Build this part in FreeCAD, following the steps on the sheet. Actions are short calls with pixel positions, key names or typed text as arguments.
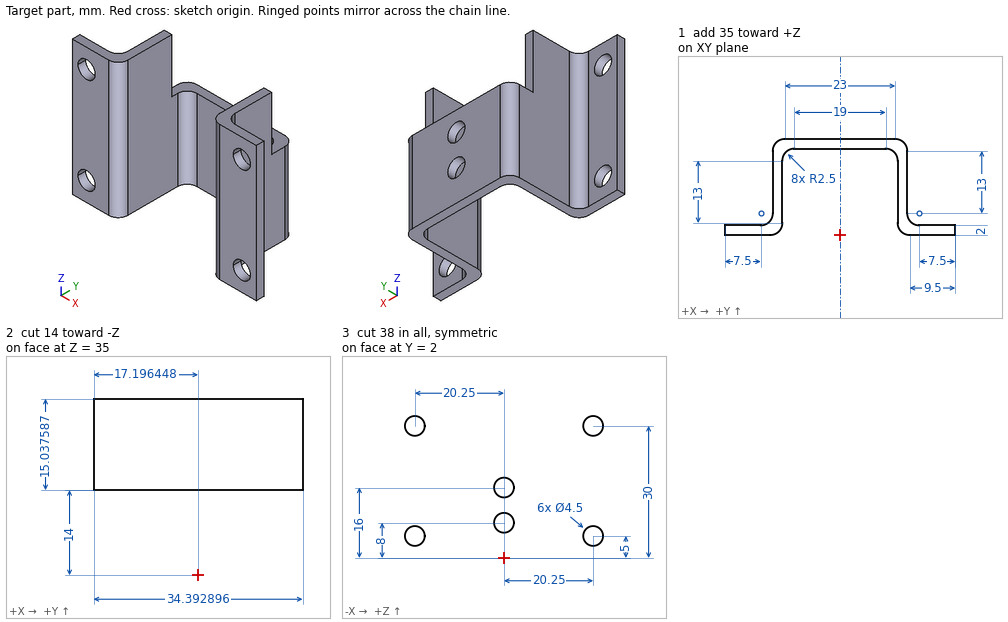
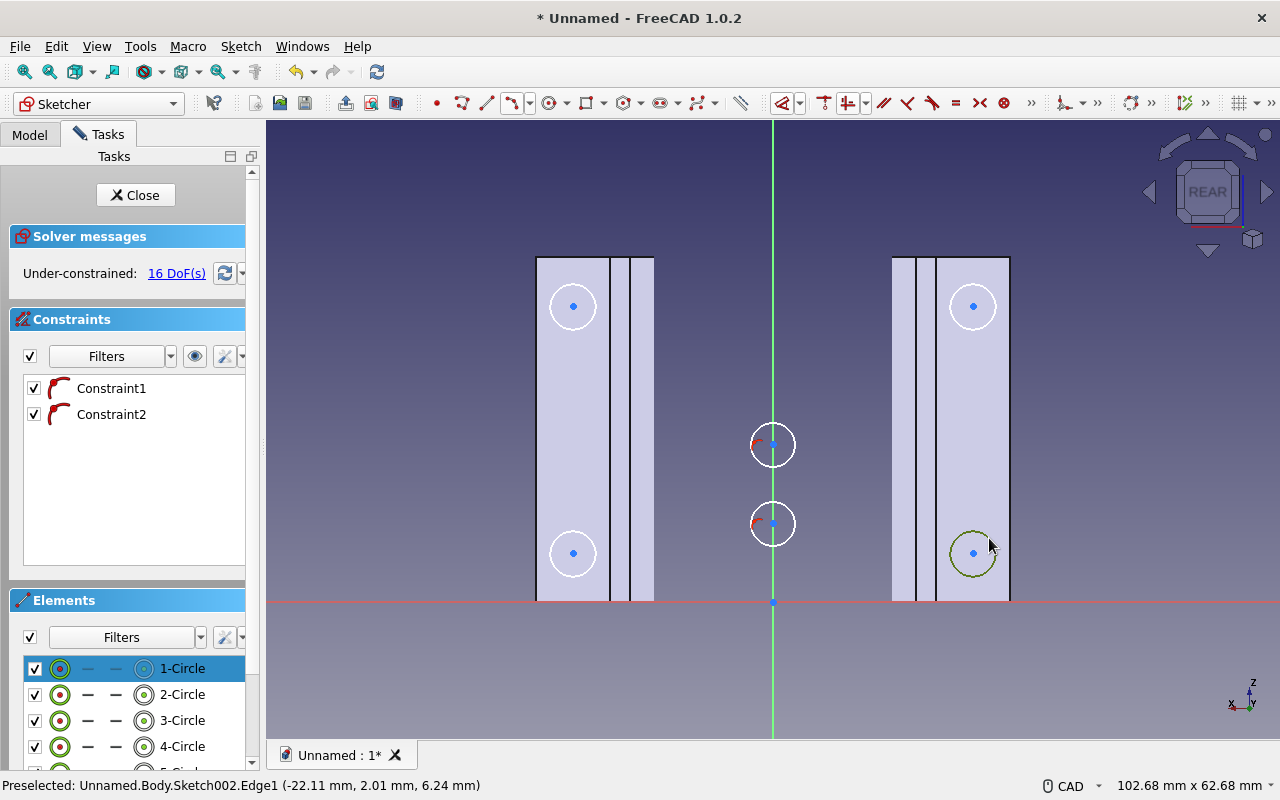
click(989, 291)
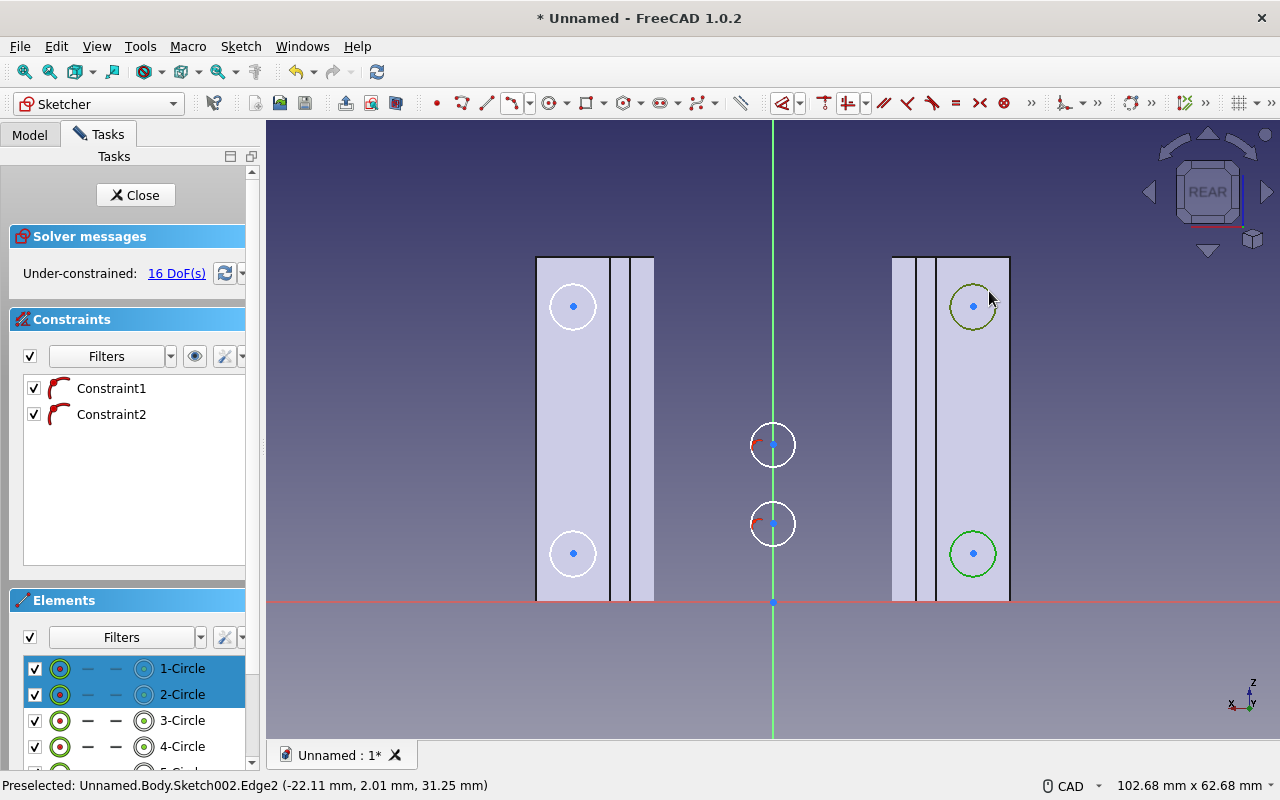
click(589, 291)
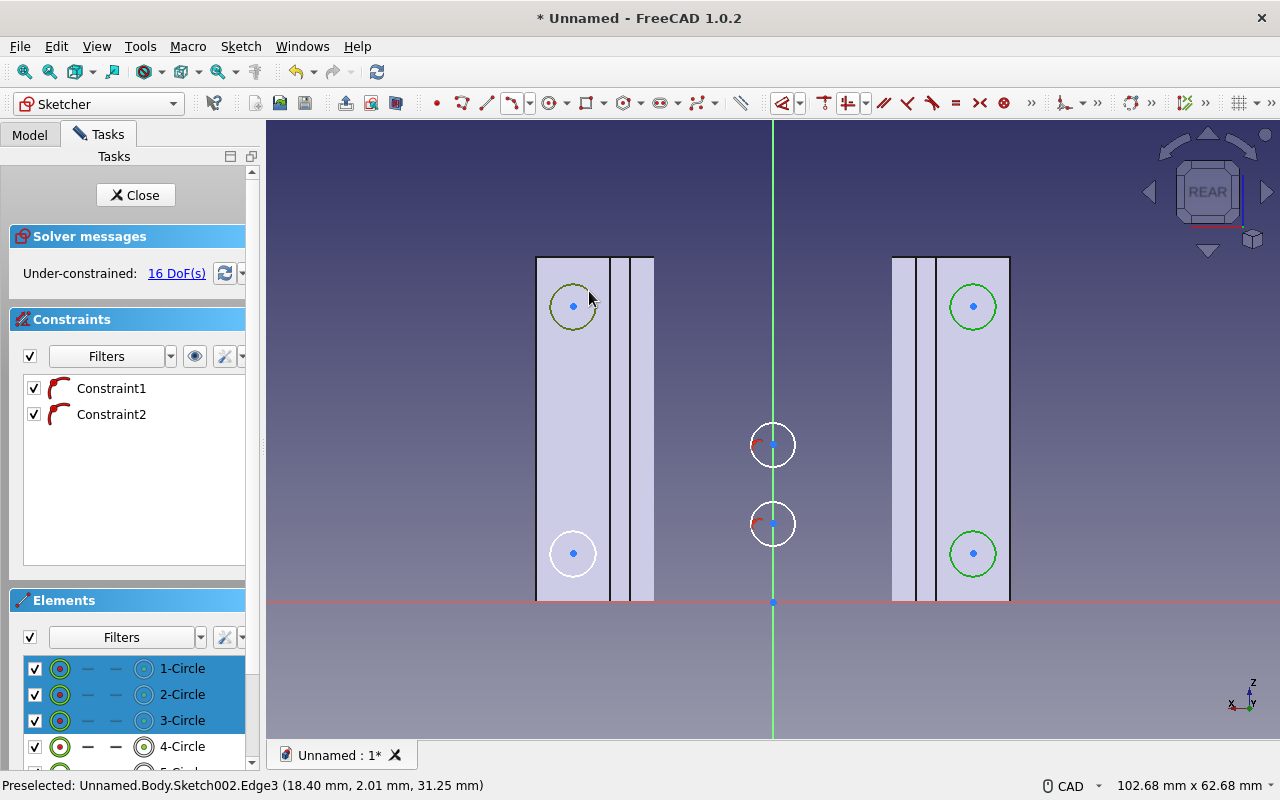
click(589, 538)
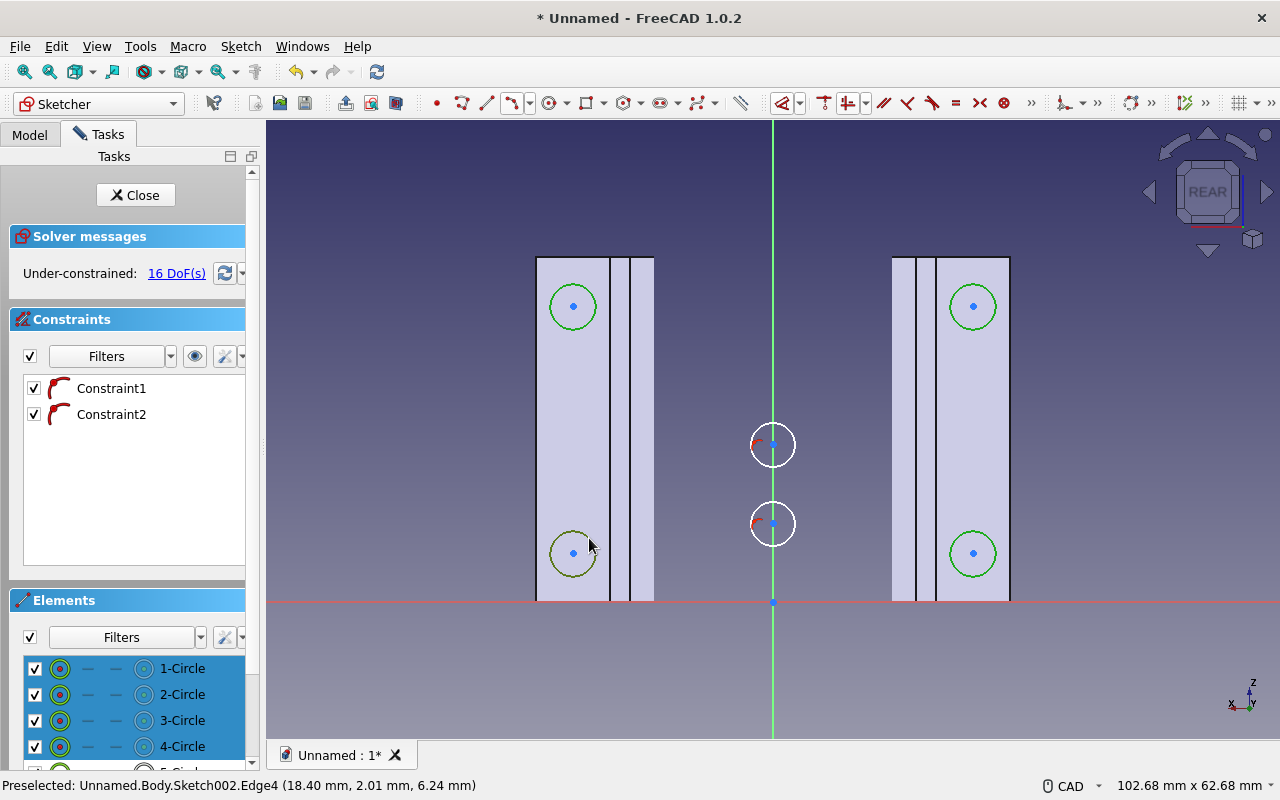
click(788, 508)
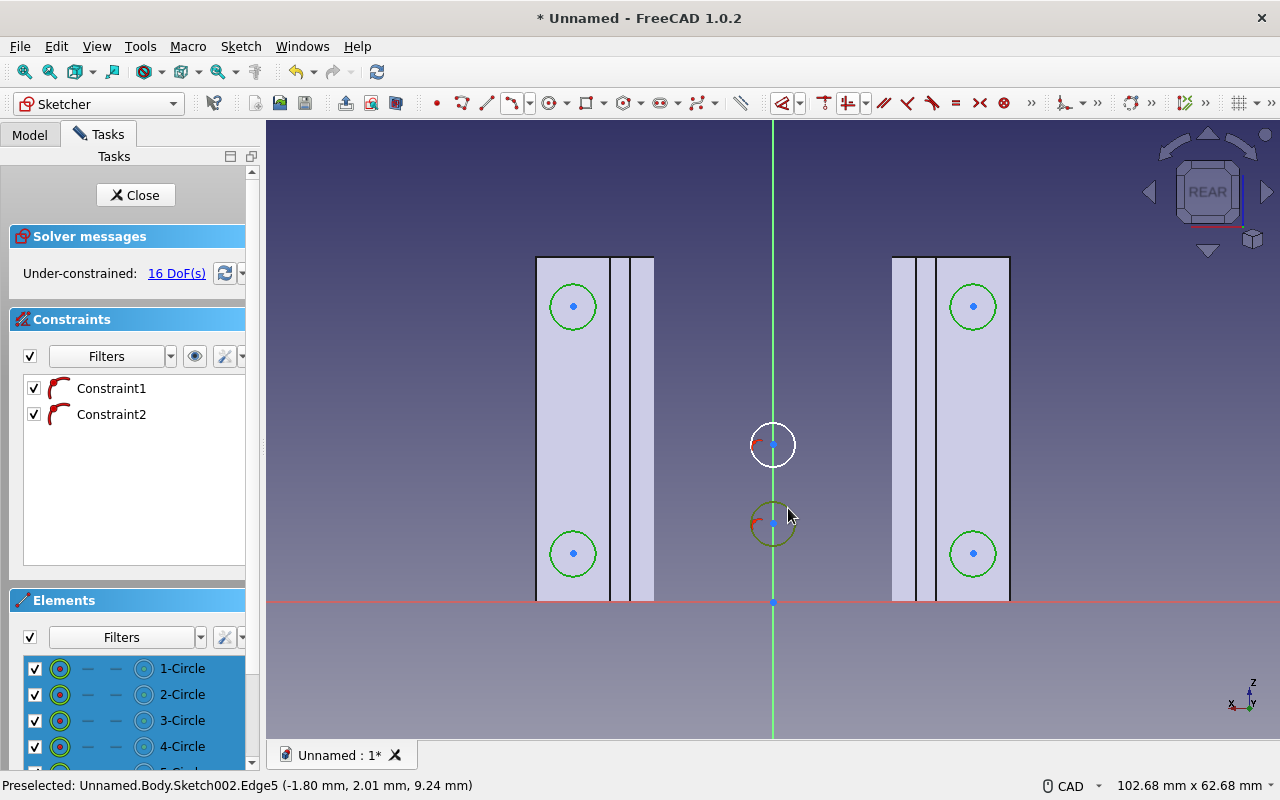
click(788, 429)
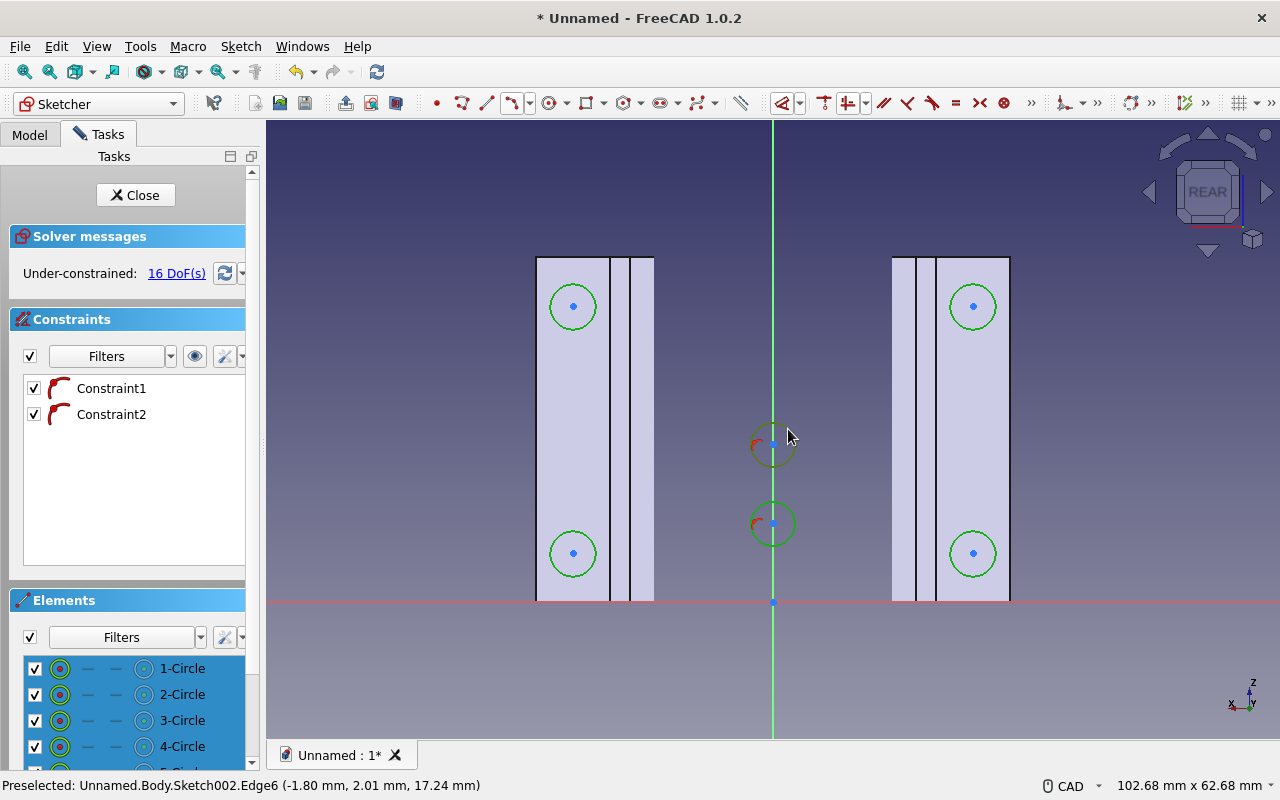
click(956, 104)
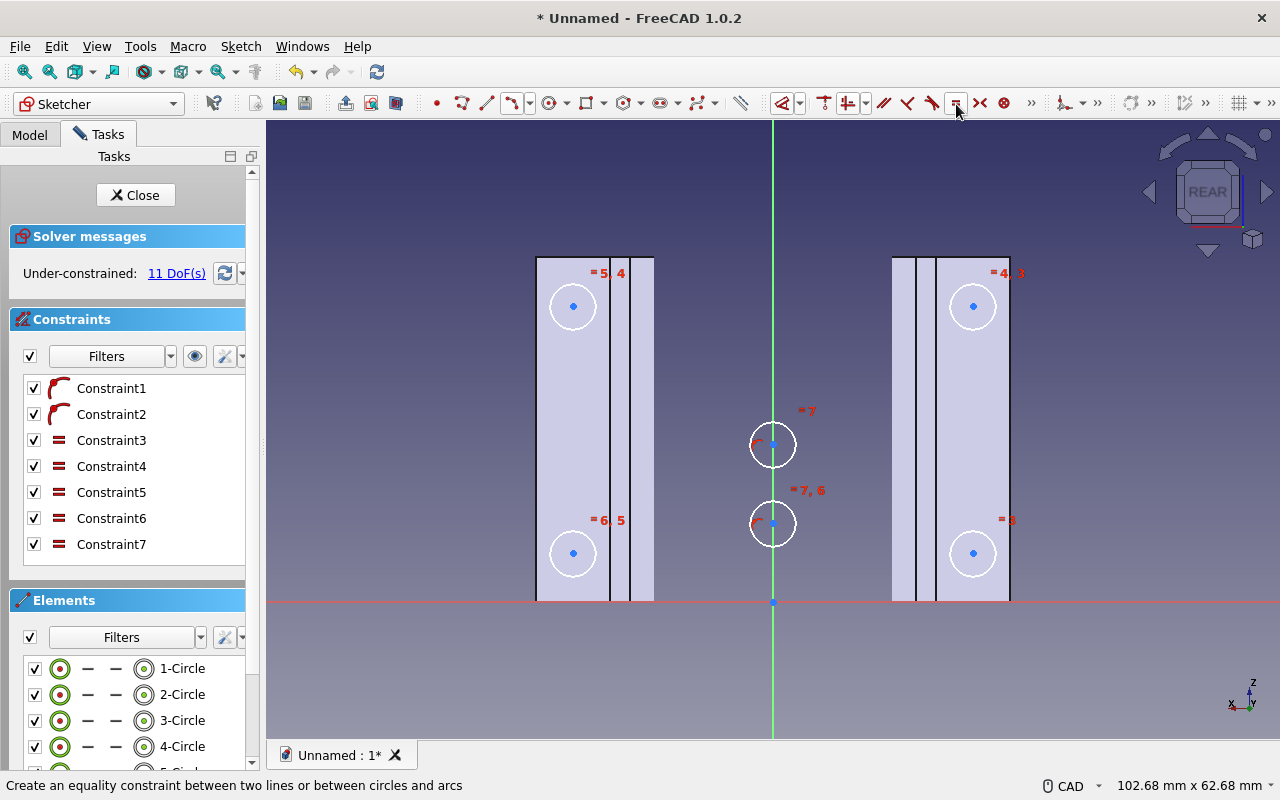
click(973, 554)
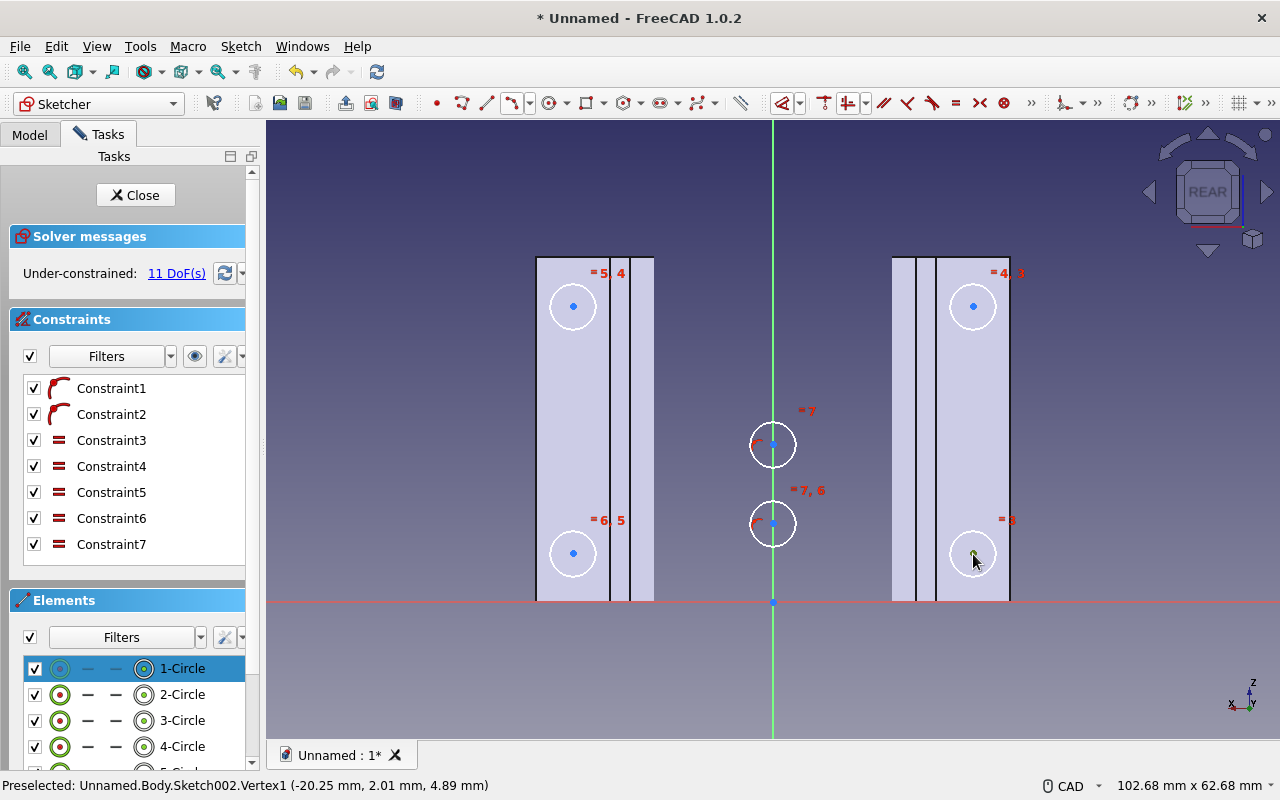
click(973, 307)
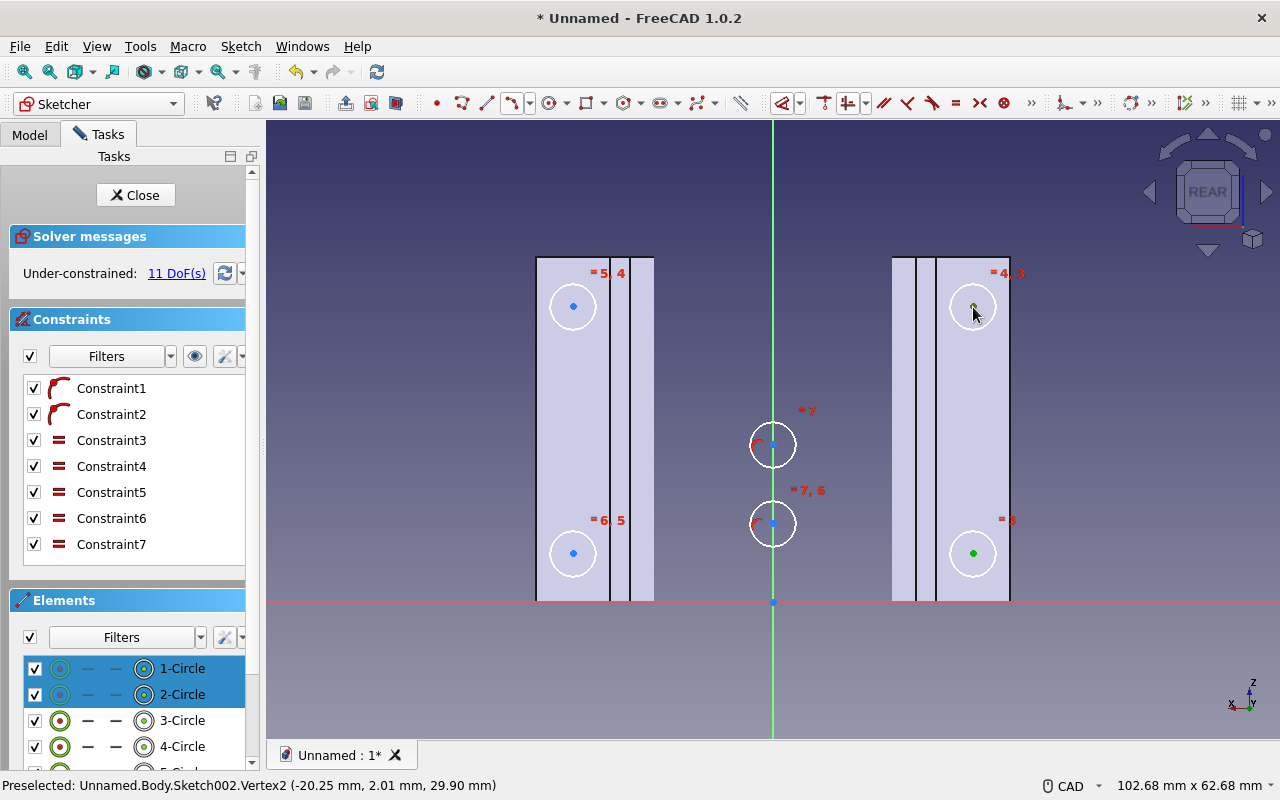
click(866, 104)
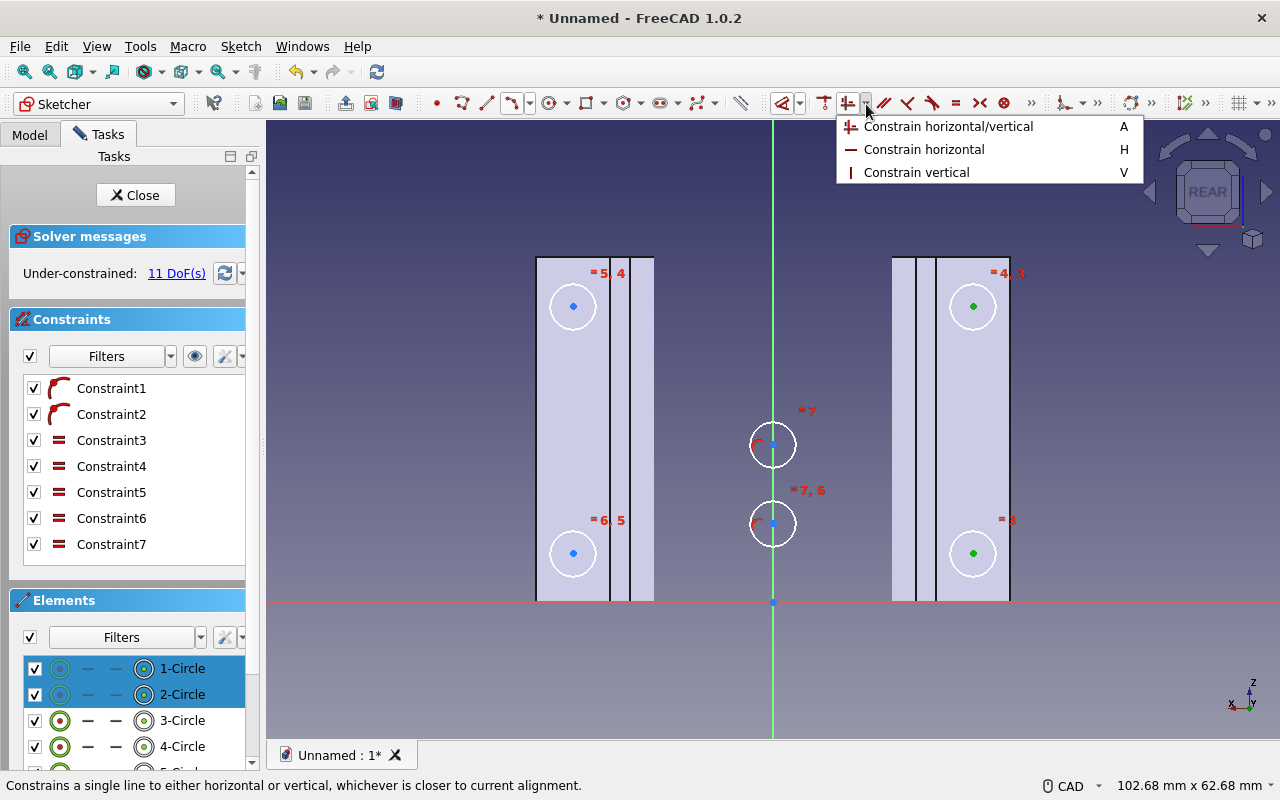
click(990, 172)